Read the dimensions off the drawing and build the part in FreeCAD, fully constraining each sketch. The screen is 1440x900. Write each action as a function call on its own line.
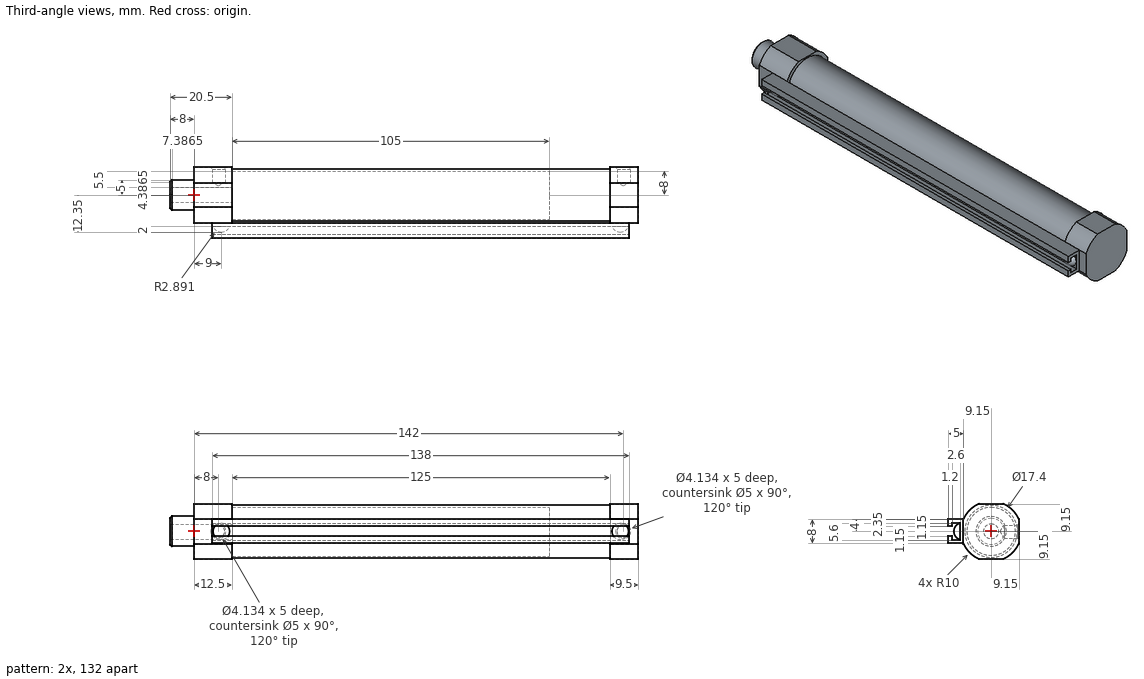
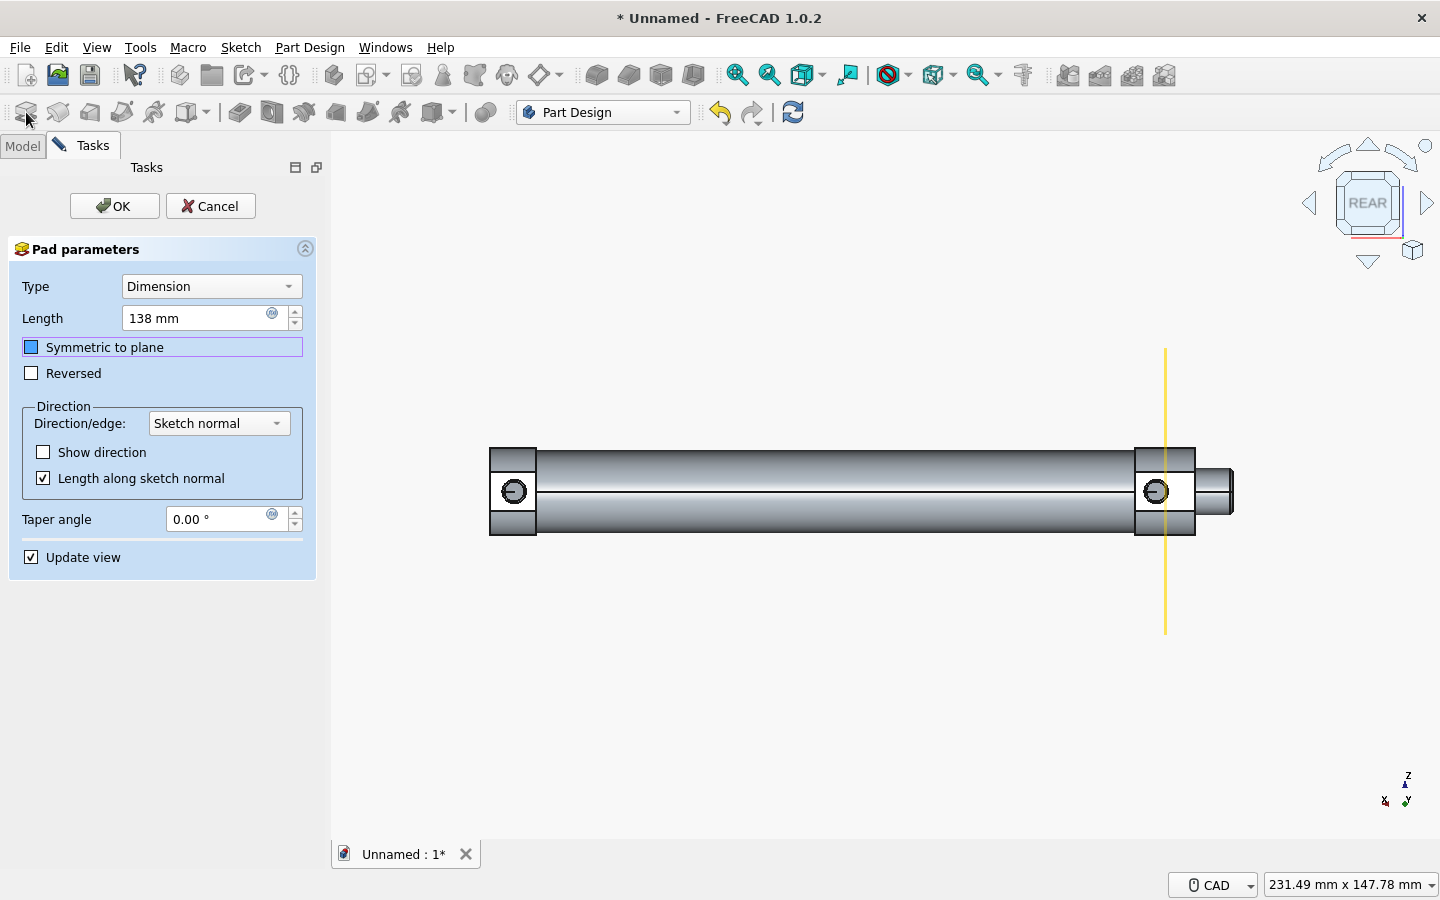
click(115, 206)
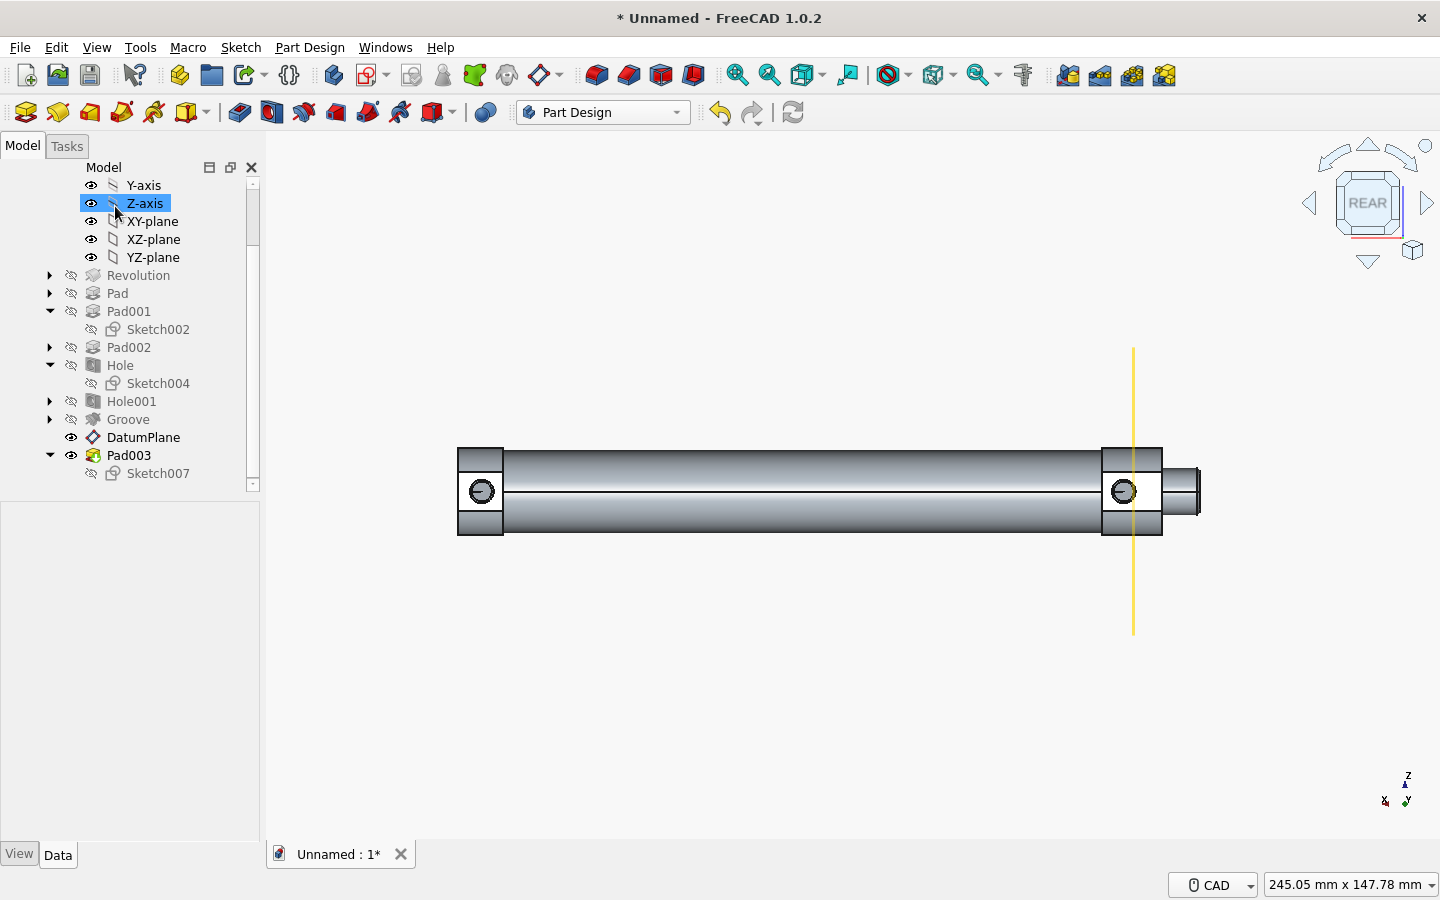
click(116, 437)
key(space)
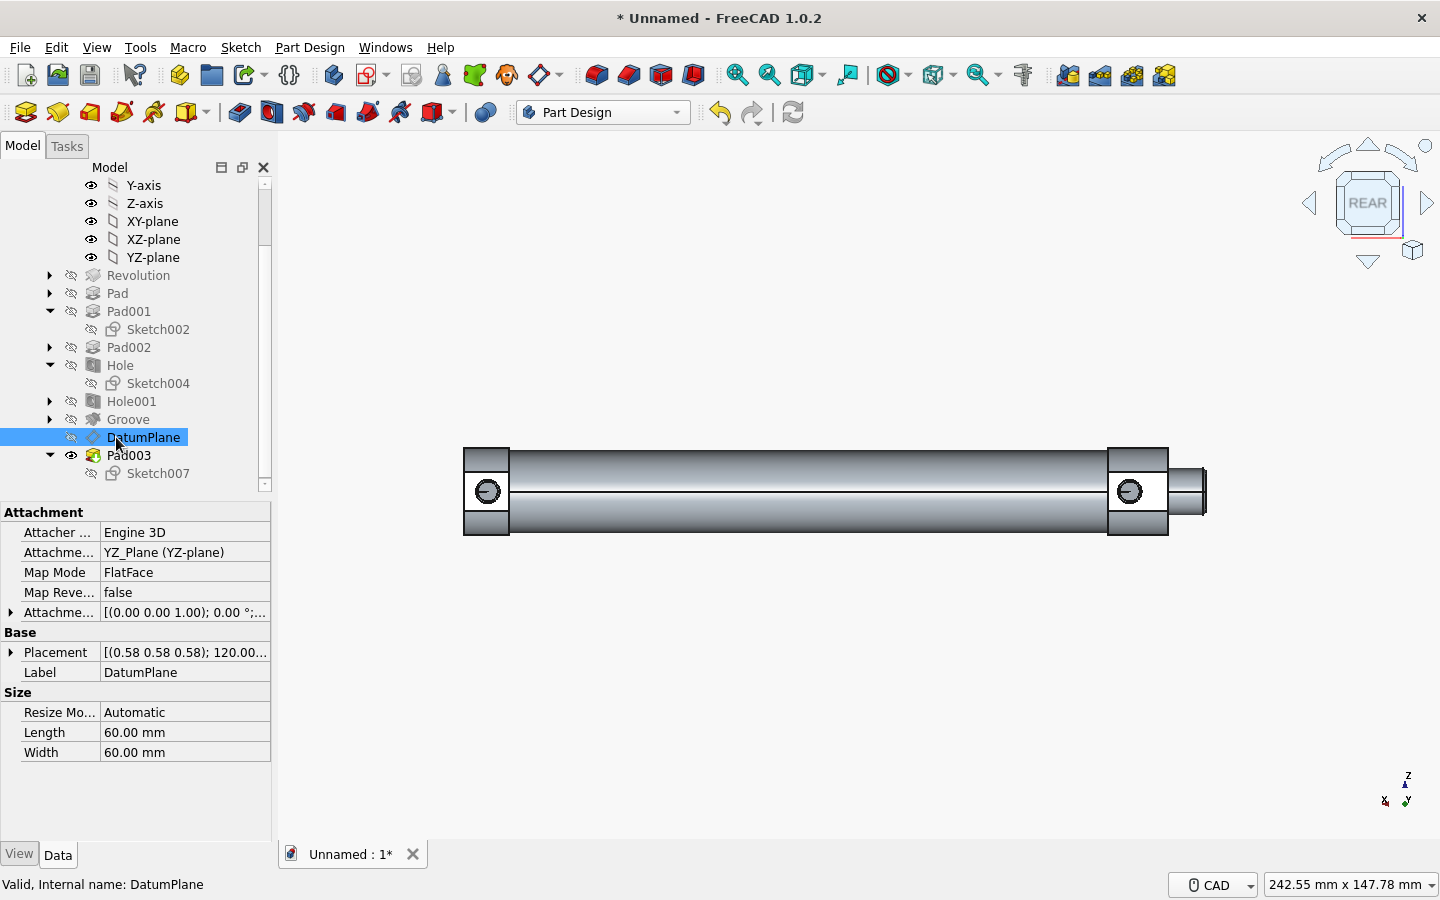
click(318, 799)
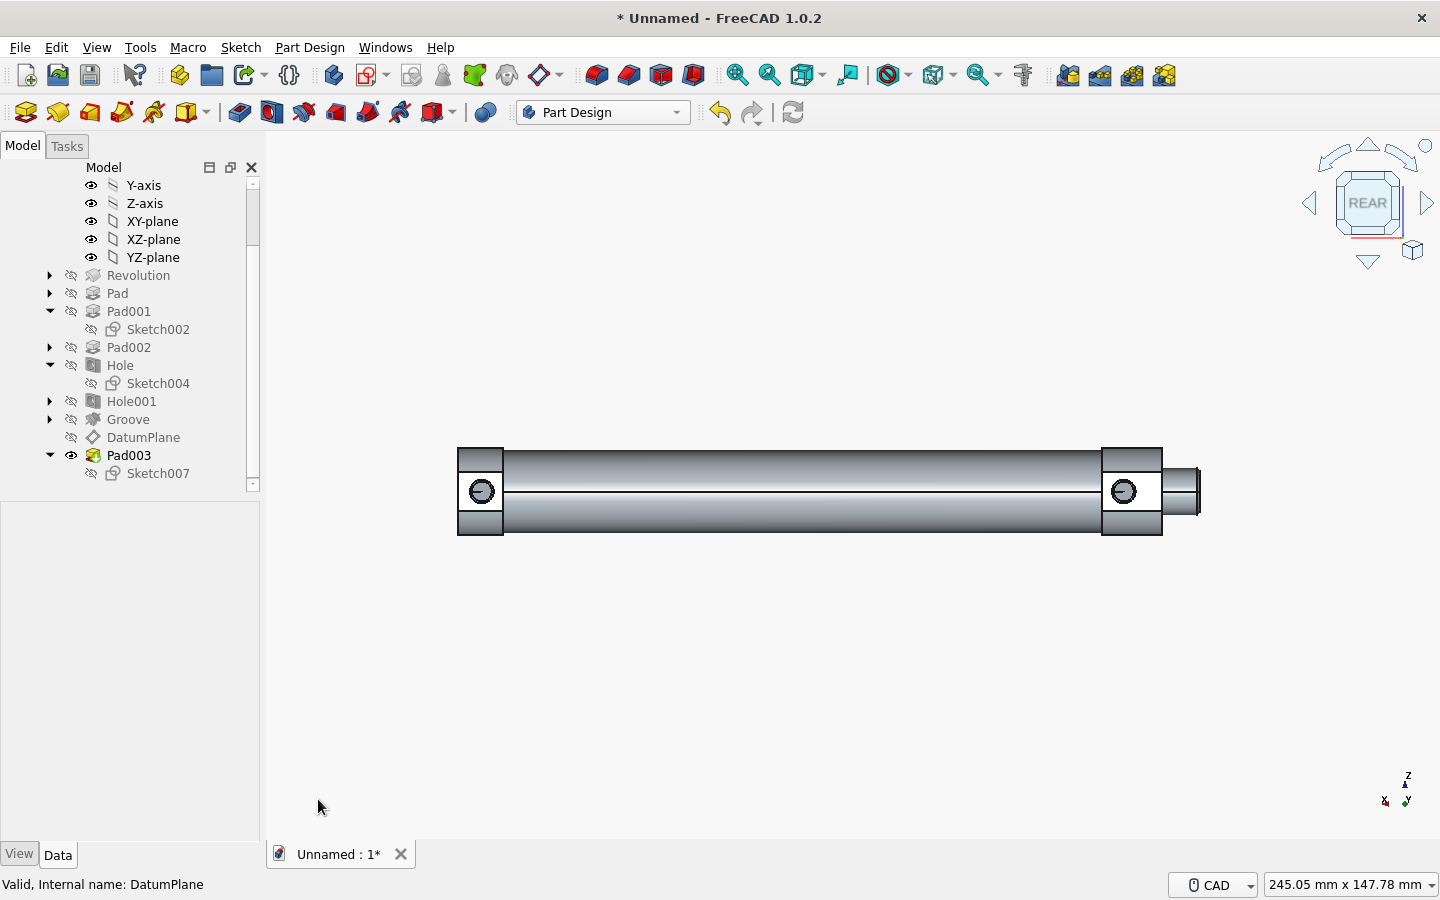
click(366, 76)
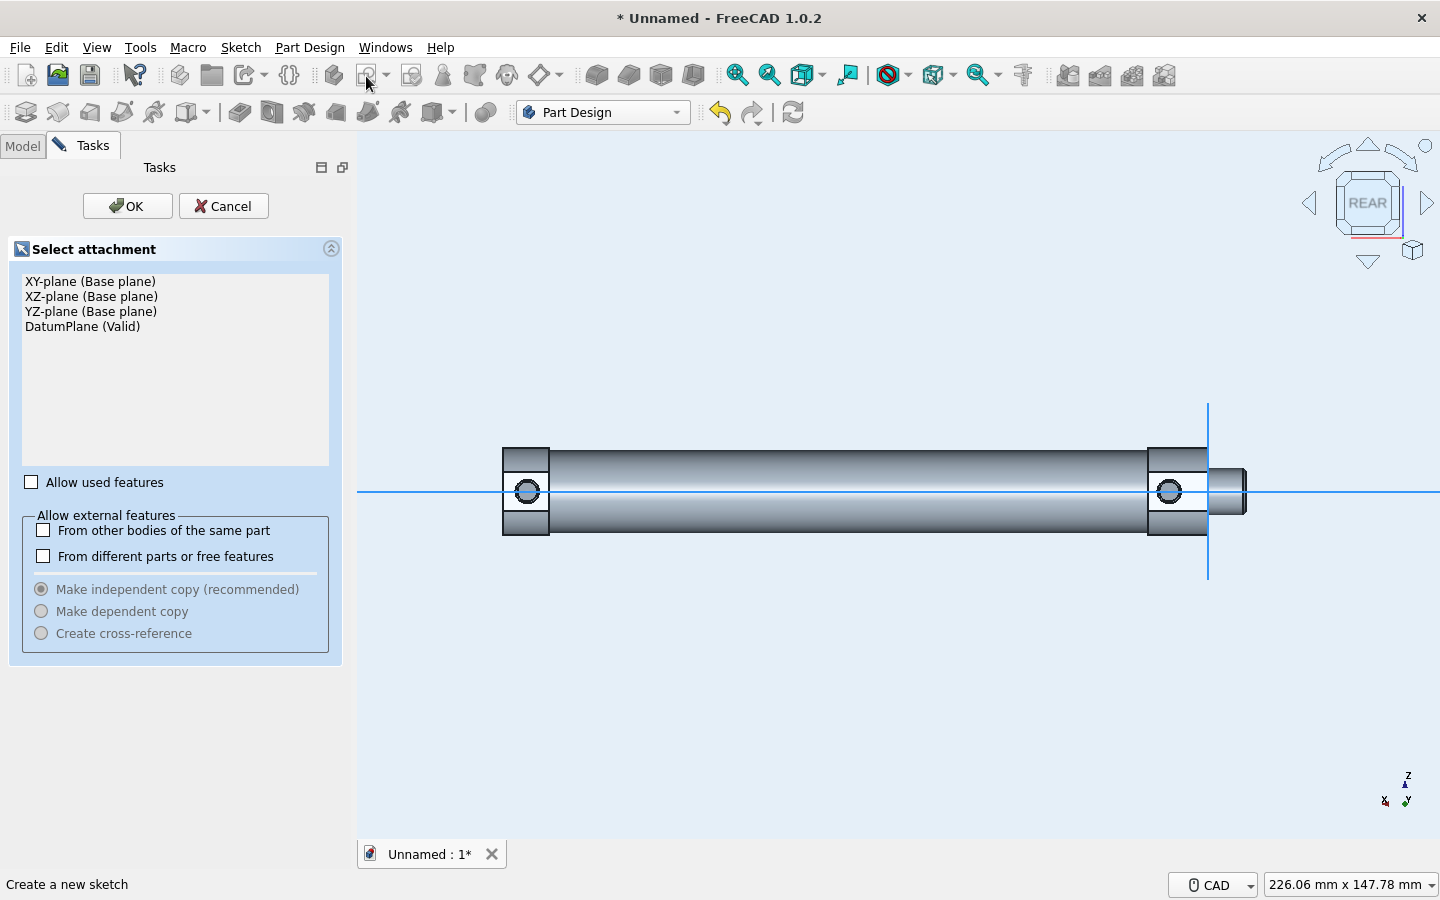
click(82, 282)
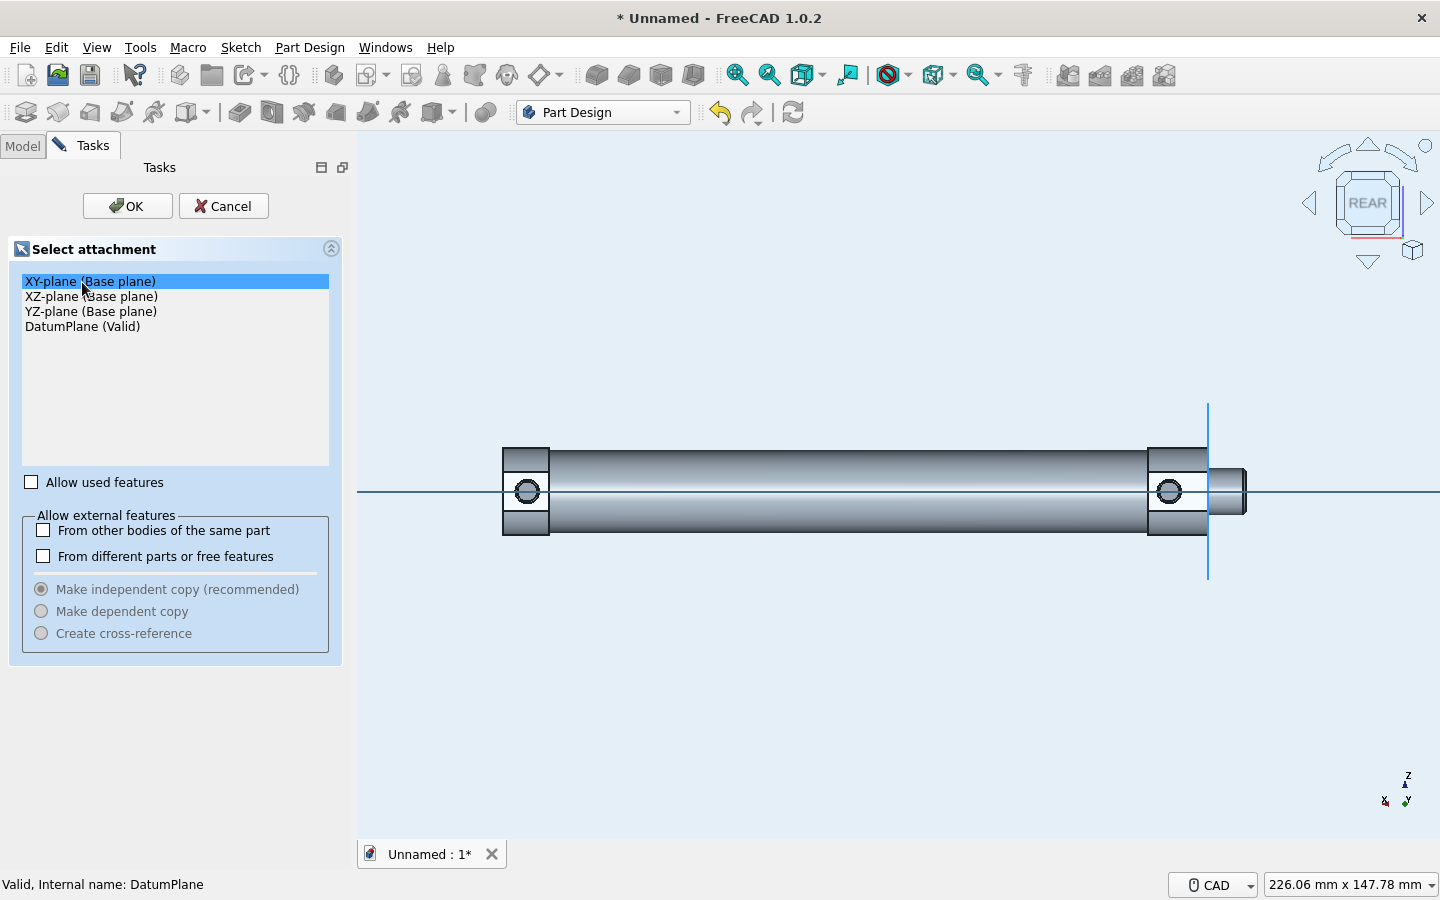
click(128, 206)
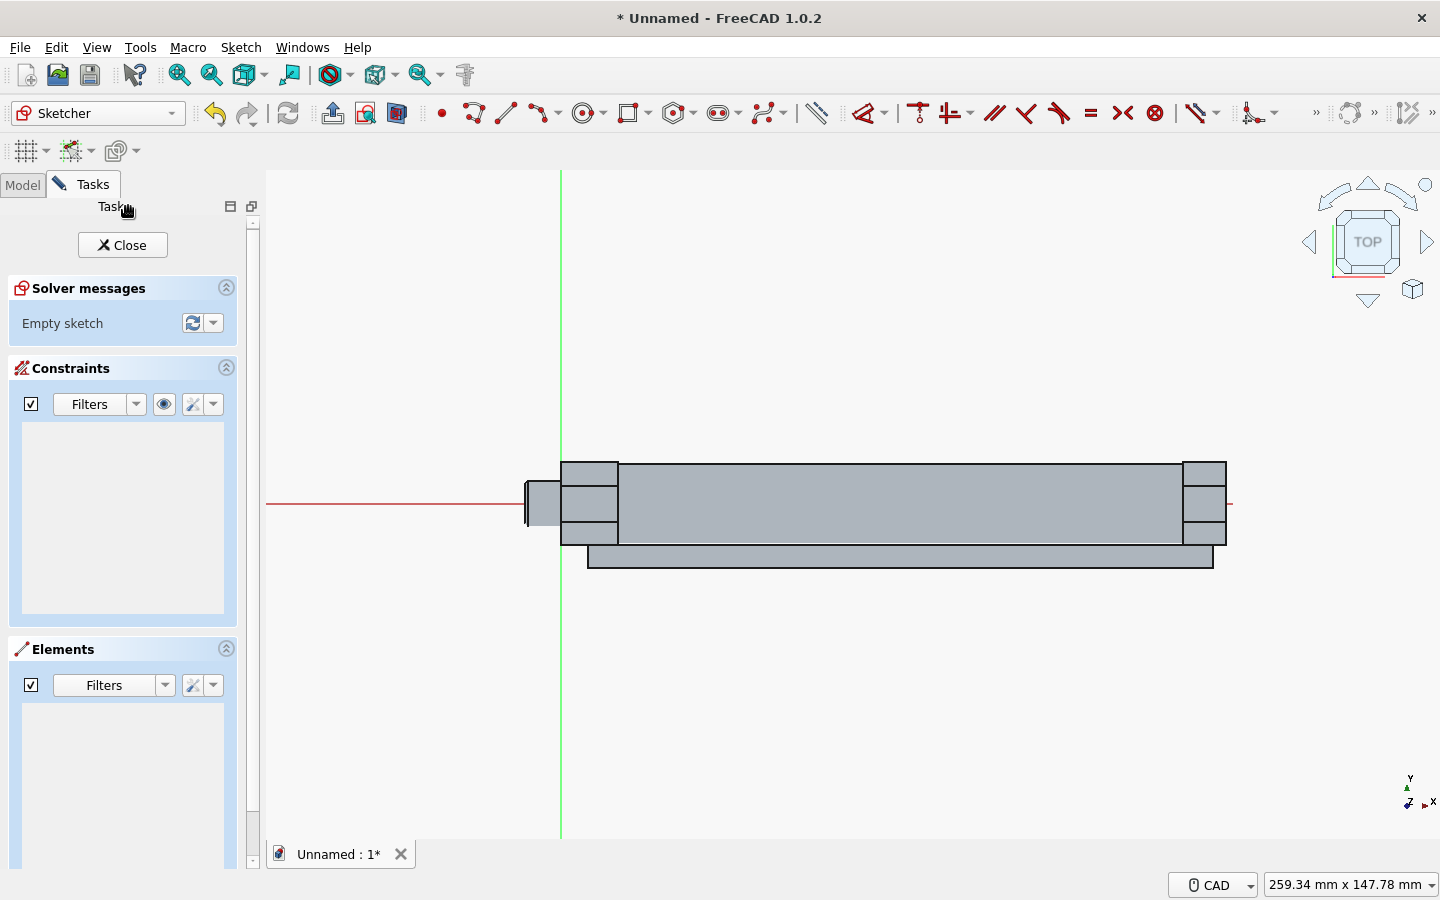
click(398, 114)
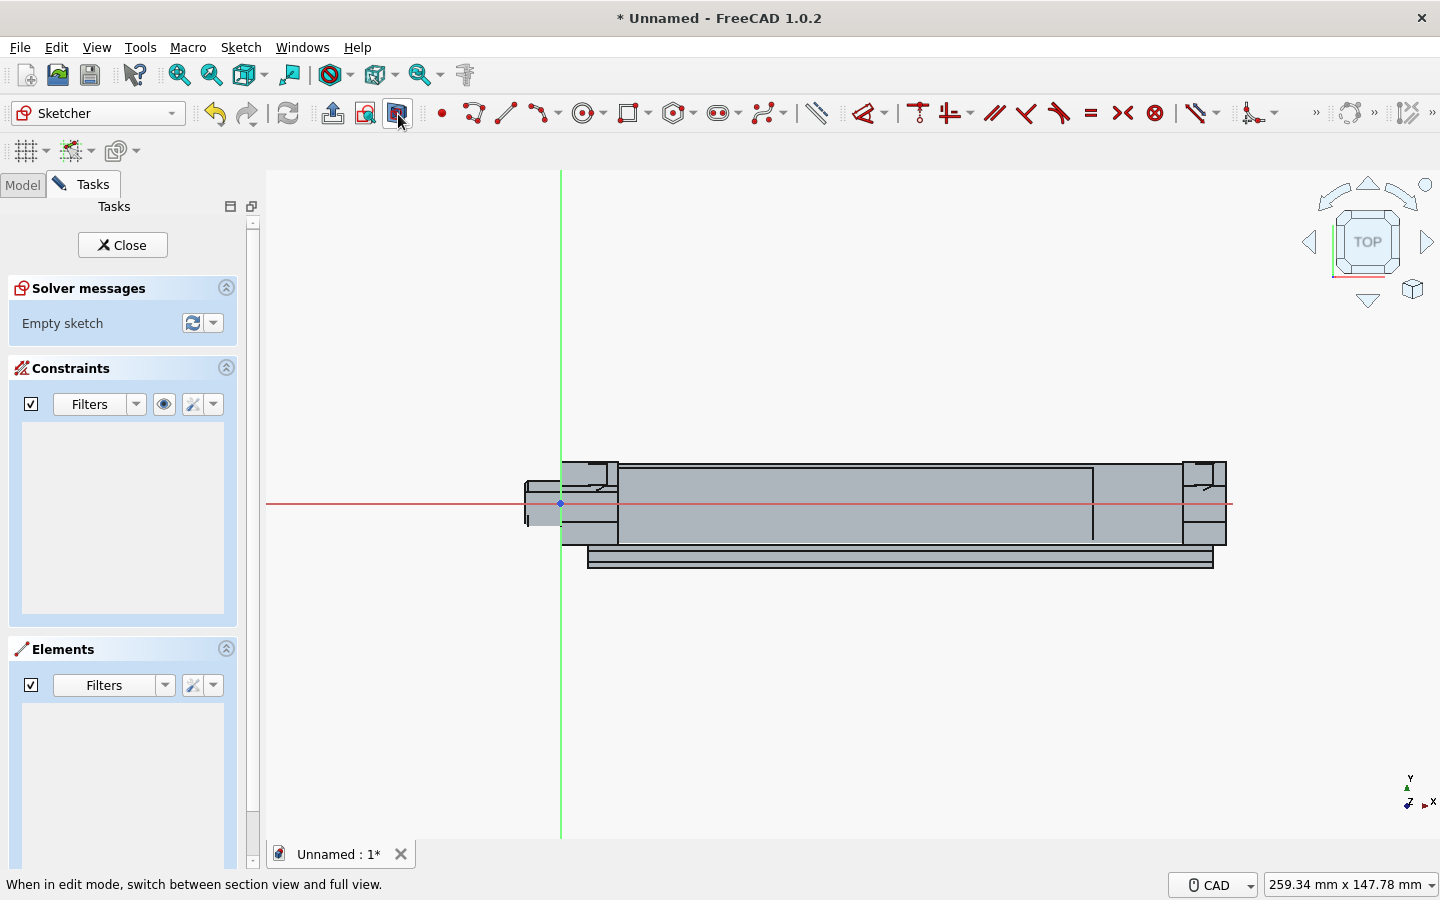
scroll(586, 560, up, 15)